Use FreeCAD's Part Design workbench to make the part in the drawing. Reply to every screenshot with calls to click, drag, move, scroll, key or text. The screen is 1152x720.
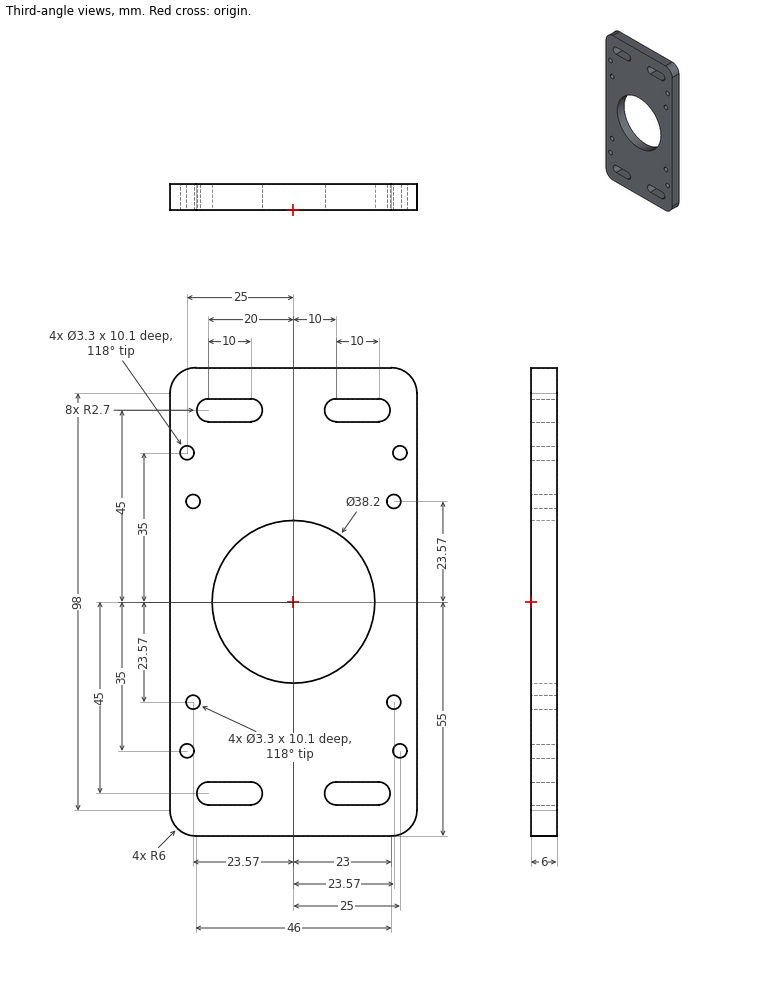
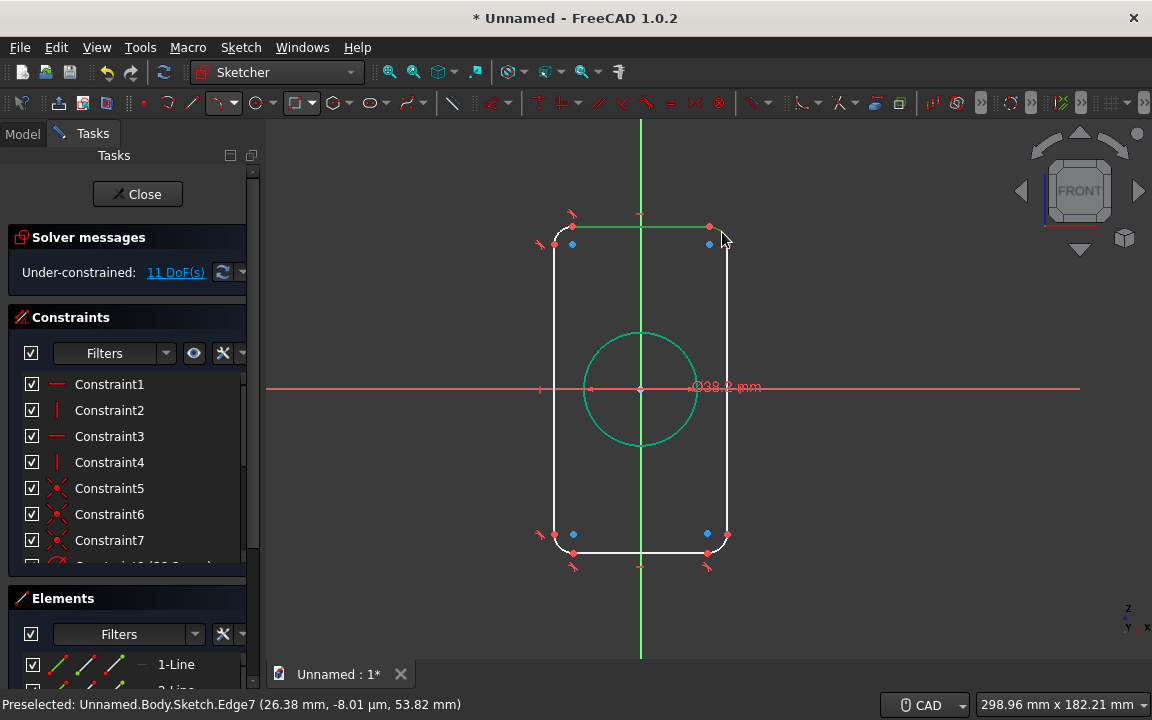
key(t)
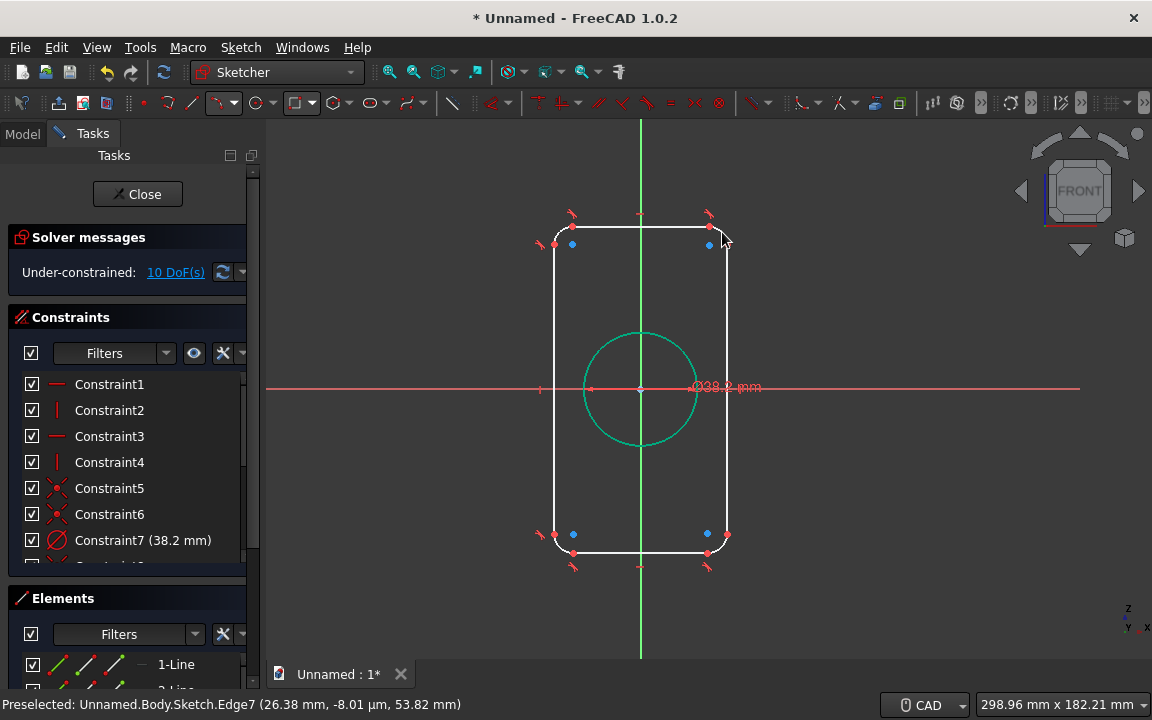
click(727, 332)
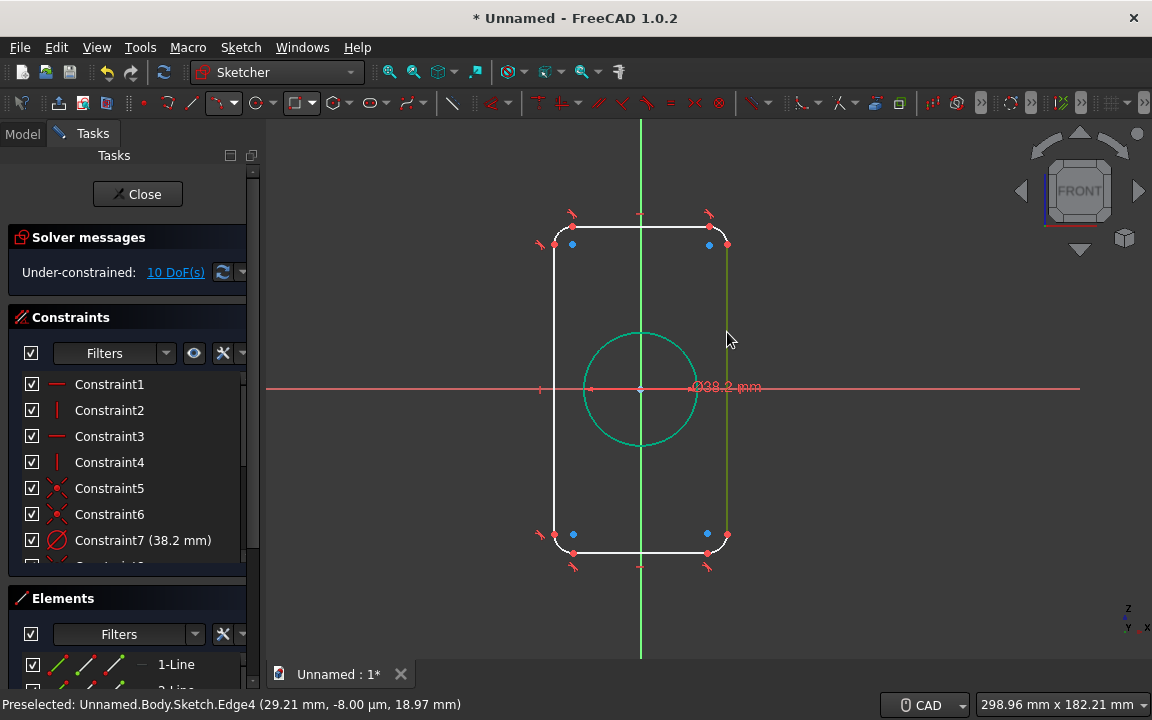
click(722, 232)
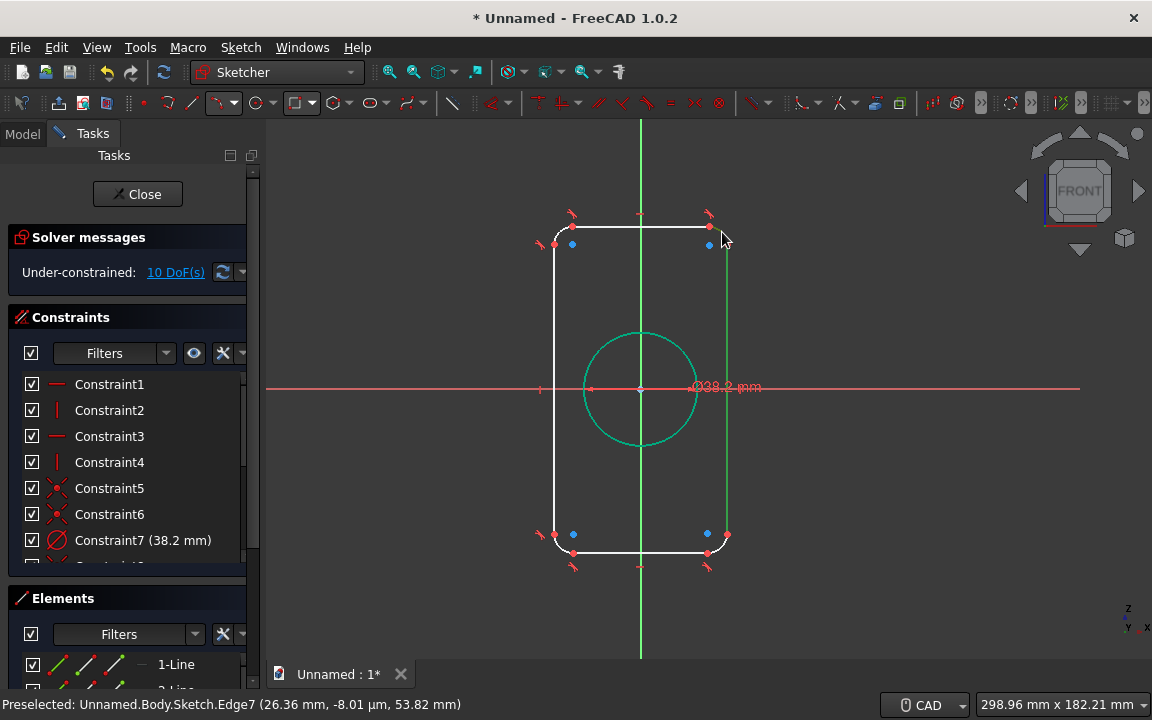
click(648, 104)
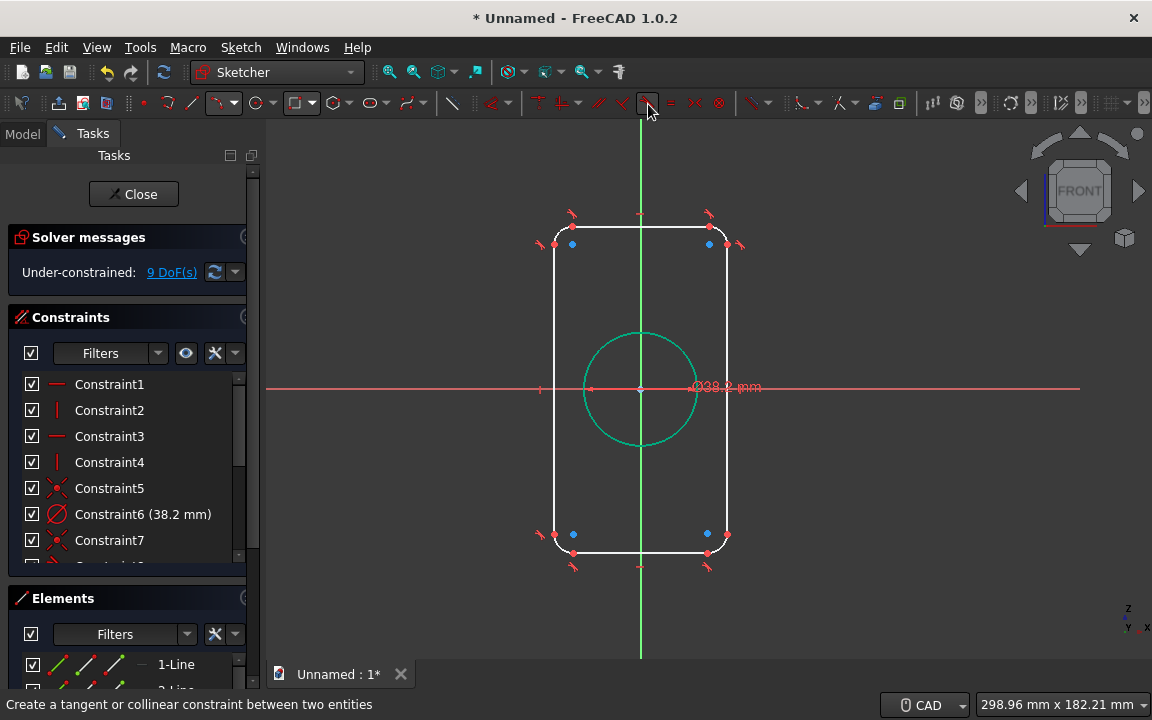
click(727, 332)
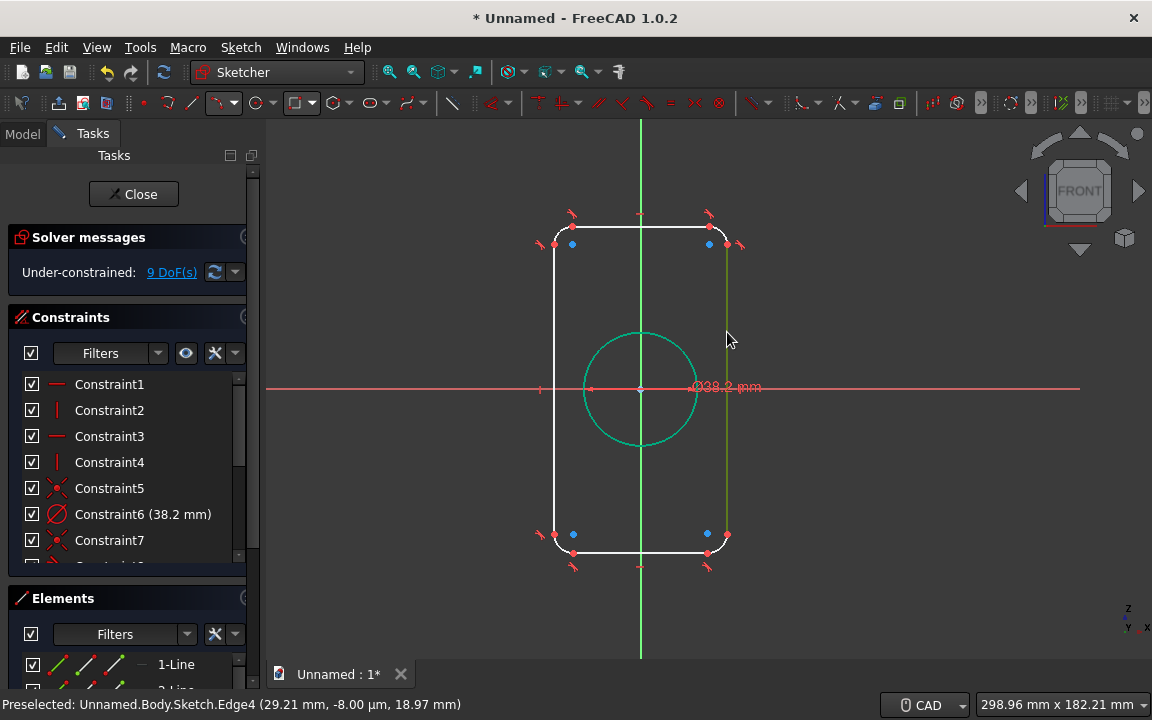
click(721, 548)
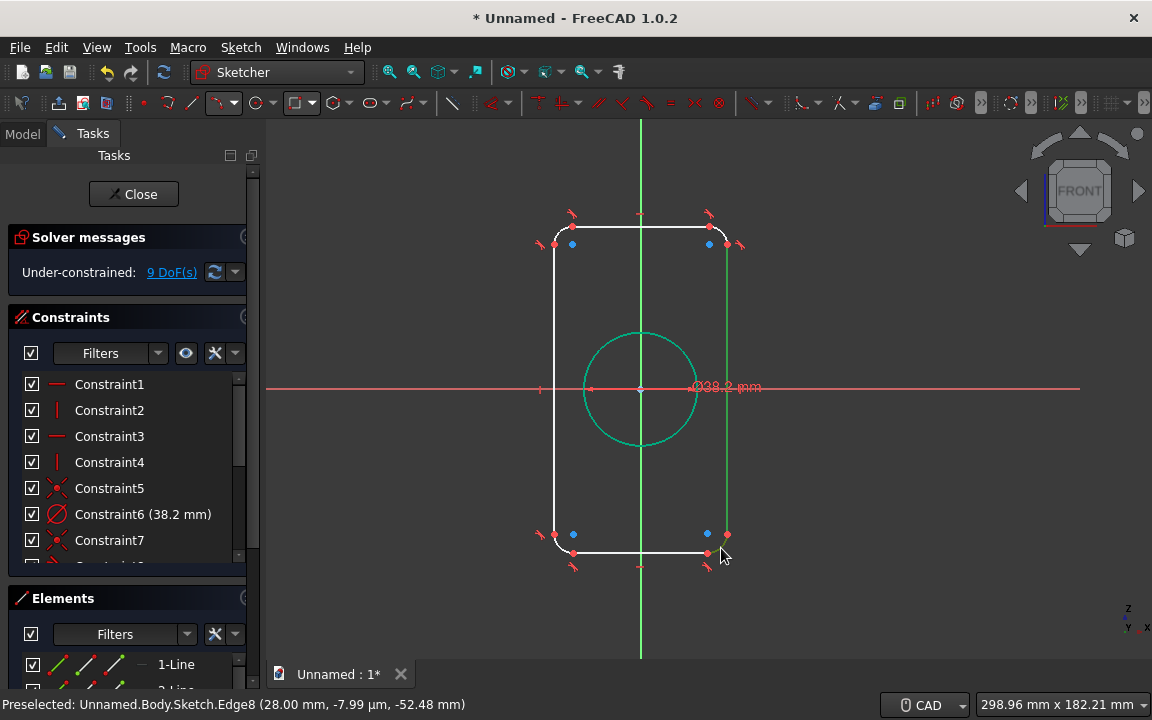
click(648, 104)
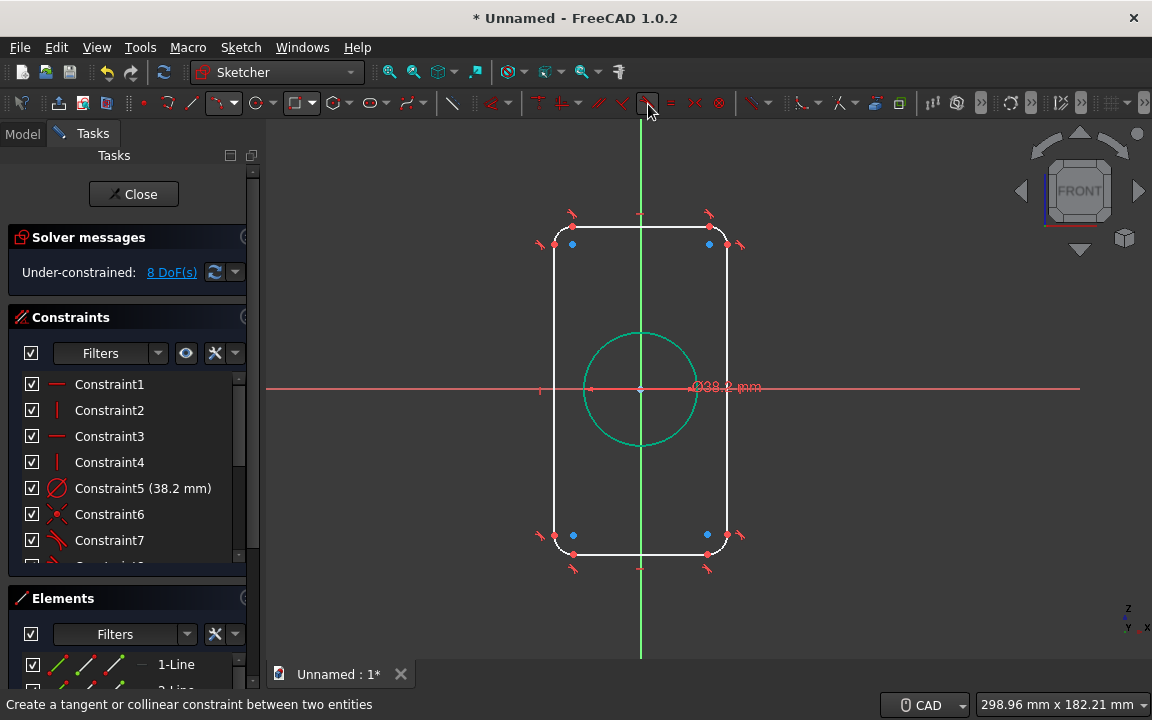
click(560, 549)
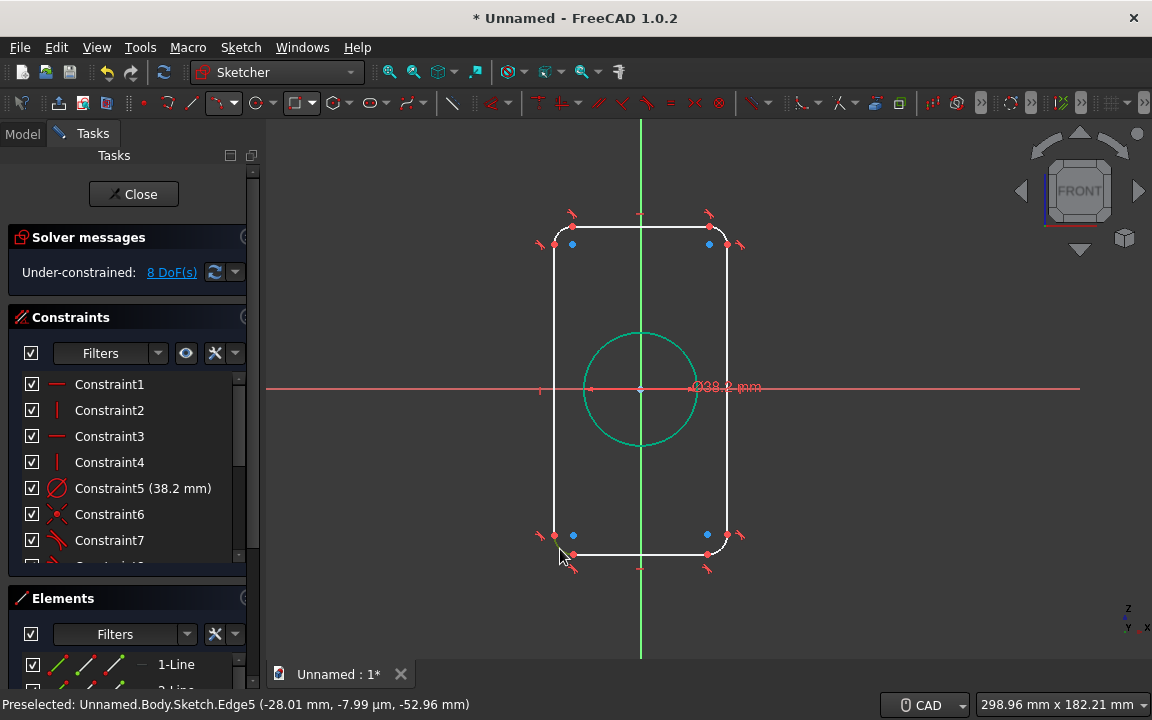
click(560, 232)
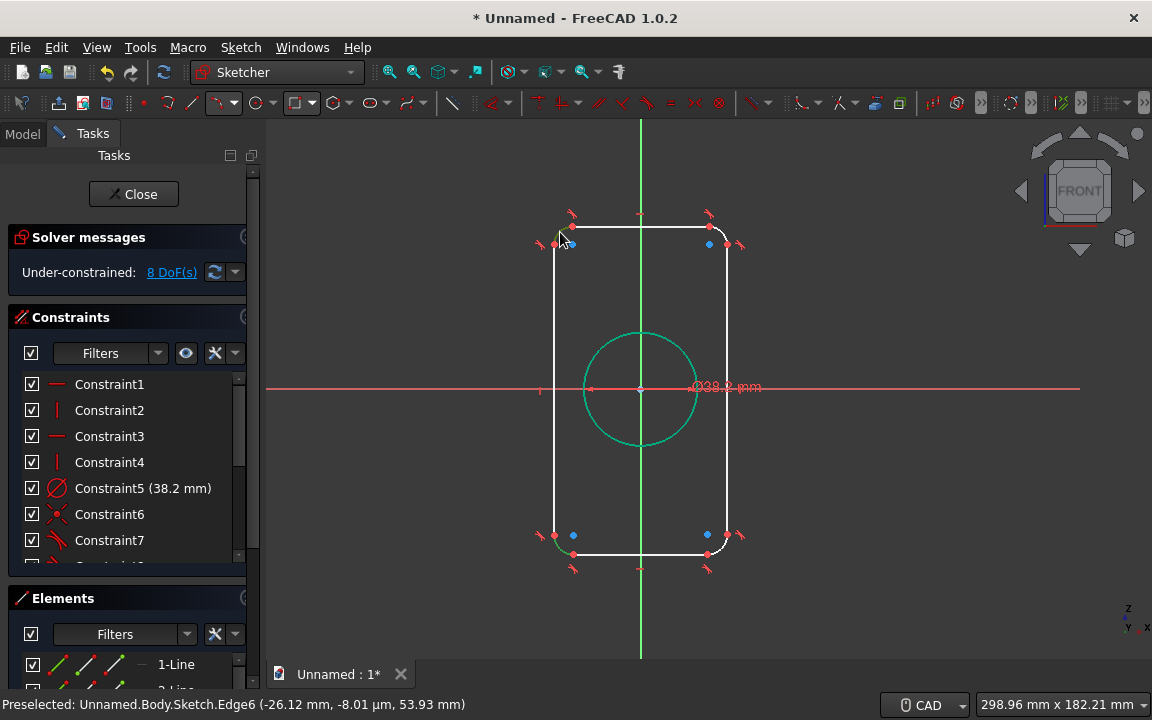
click(722, 232)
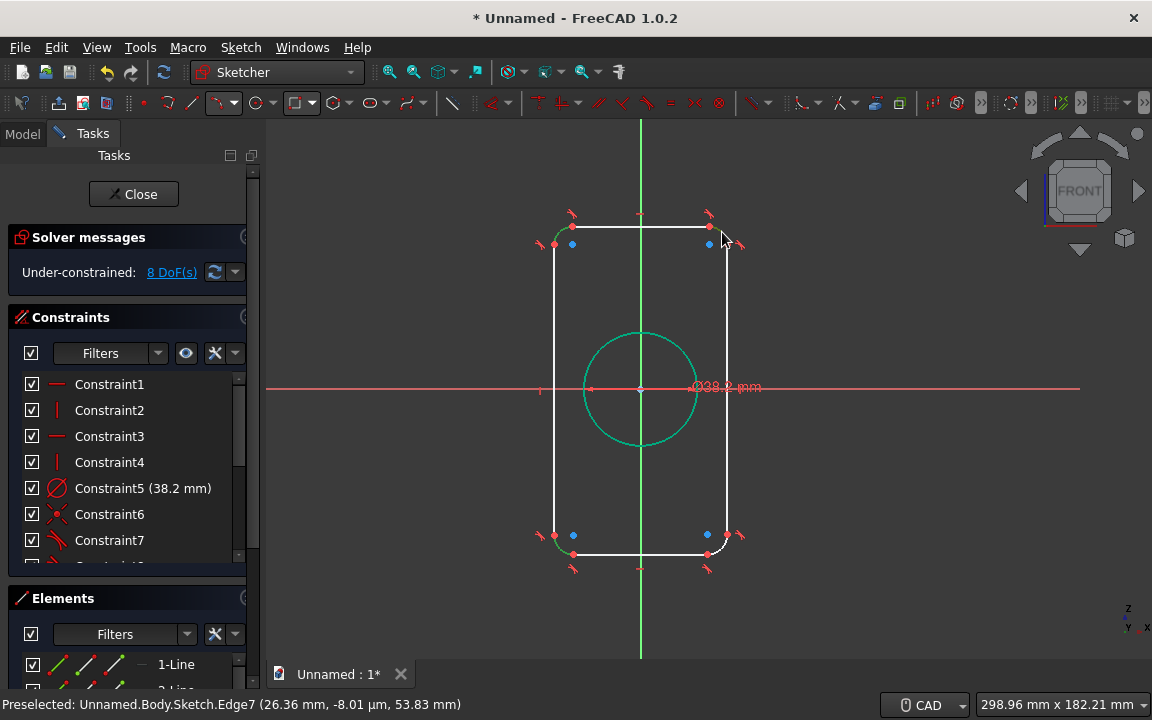
scroll(716, 552, up, 3)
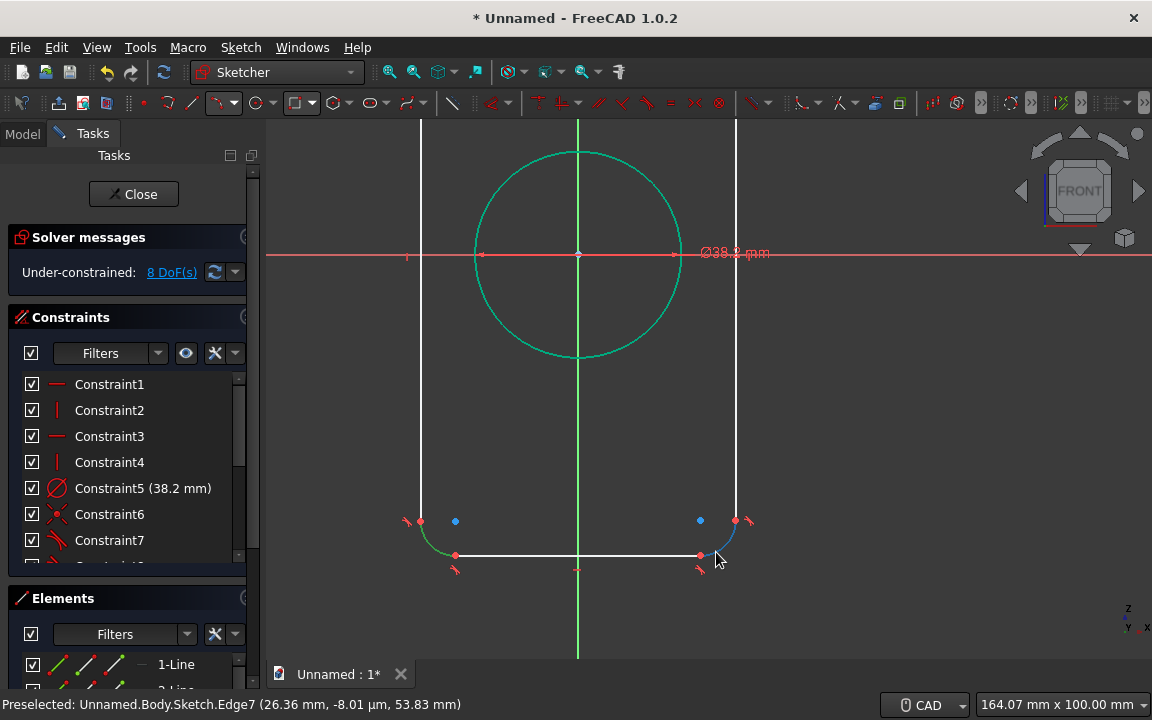
click(716, 552)